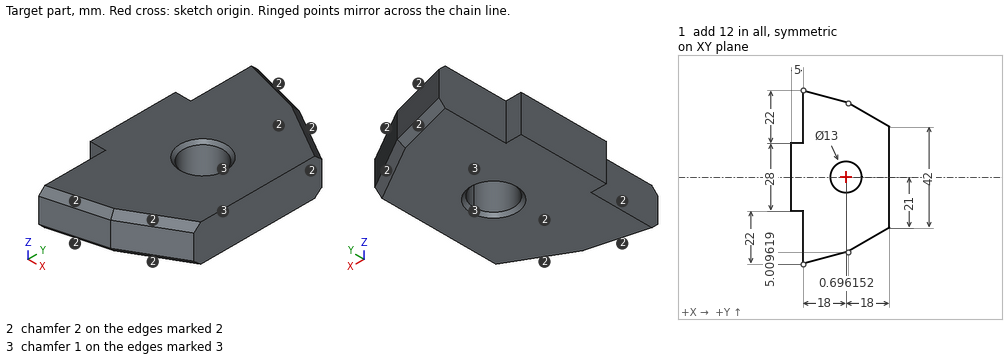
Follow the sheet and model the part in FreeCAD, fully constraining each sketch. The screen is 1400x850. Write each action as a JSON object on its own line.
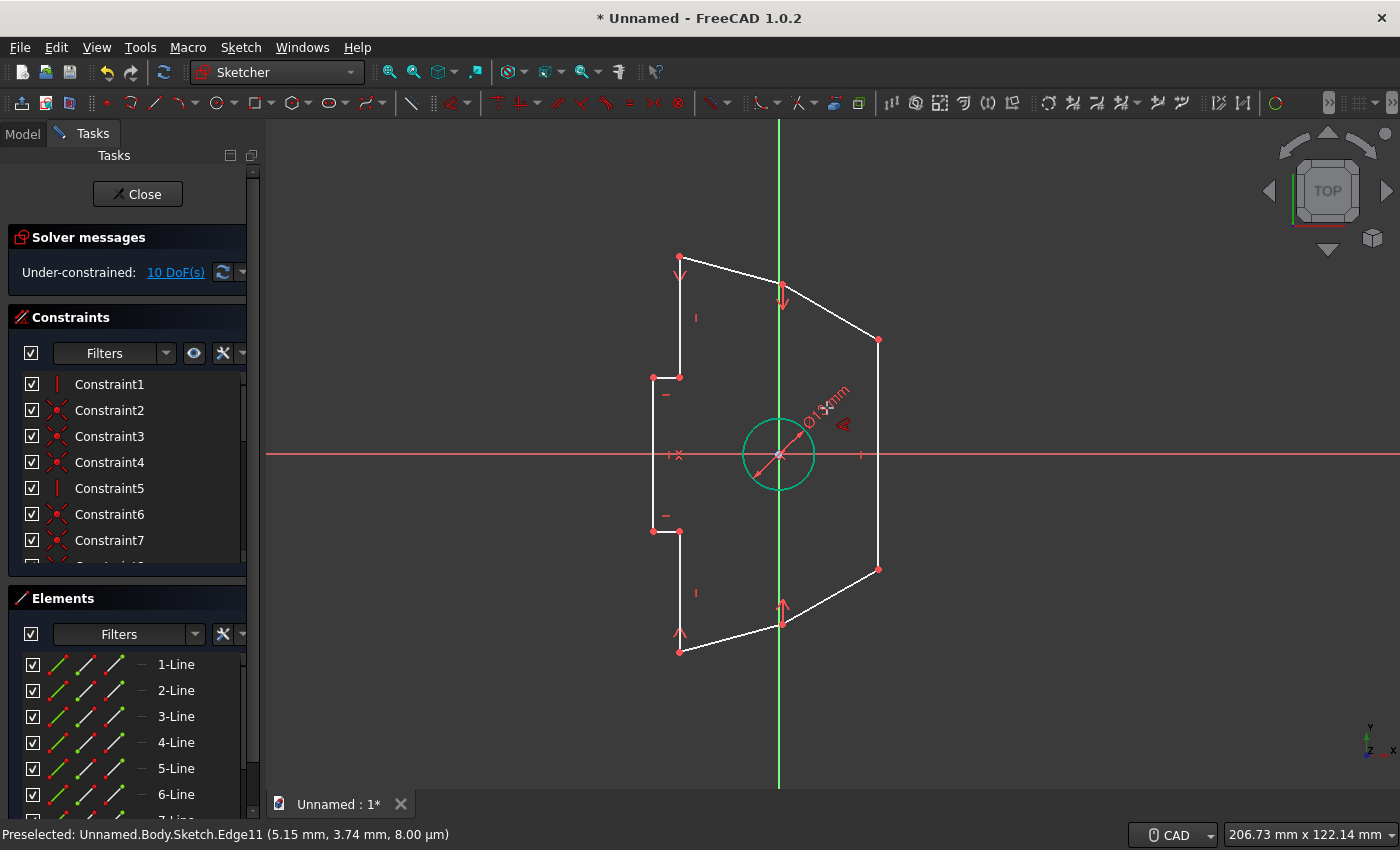
{"action": "scroll", "coordinate": [669, 378], "scroll_direction": "up", "scroll_amount": 2}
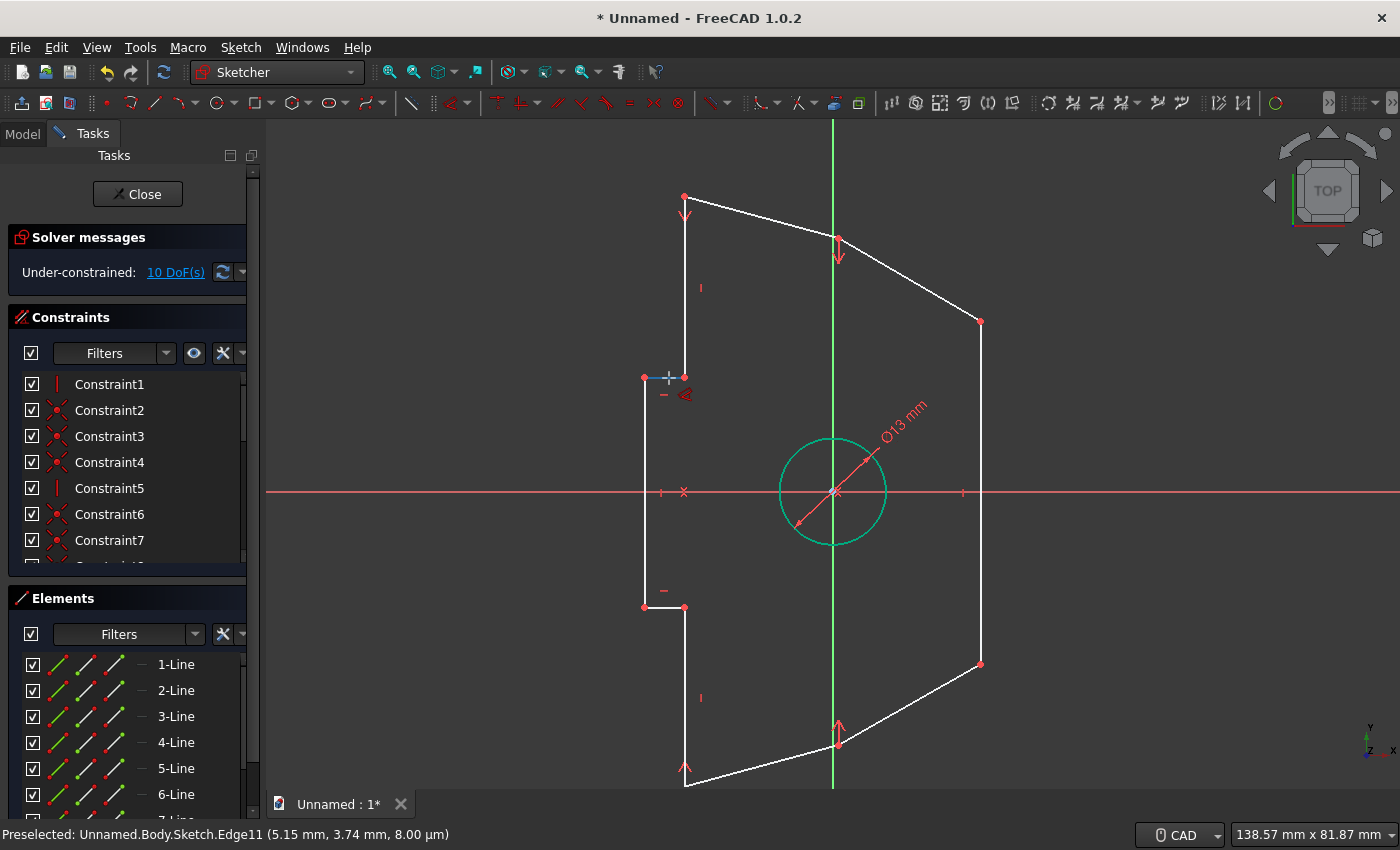
{"action": "left_click", "coordinate": [669, 378]}
{"action": "left_click", "coordinate": [665, 344]}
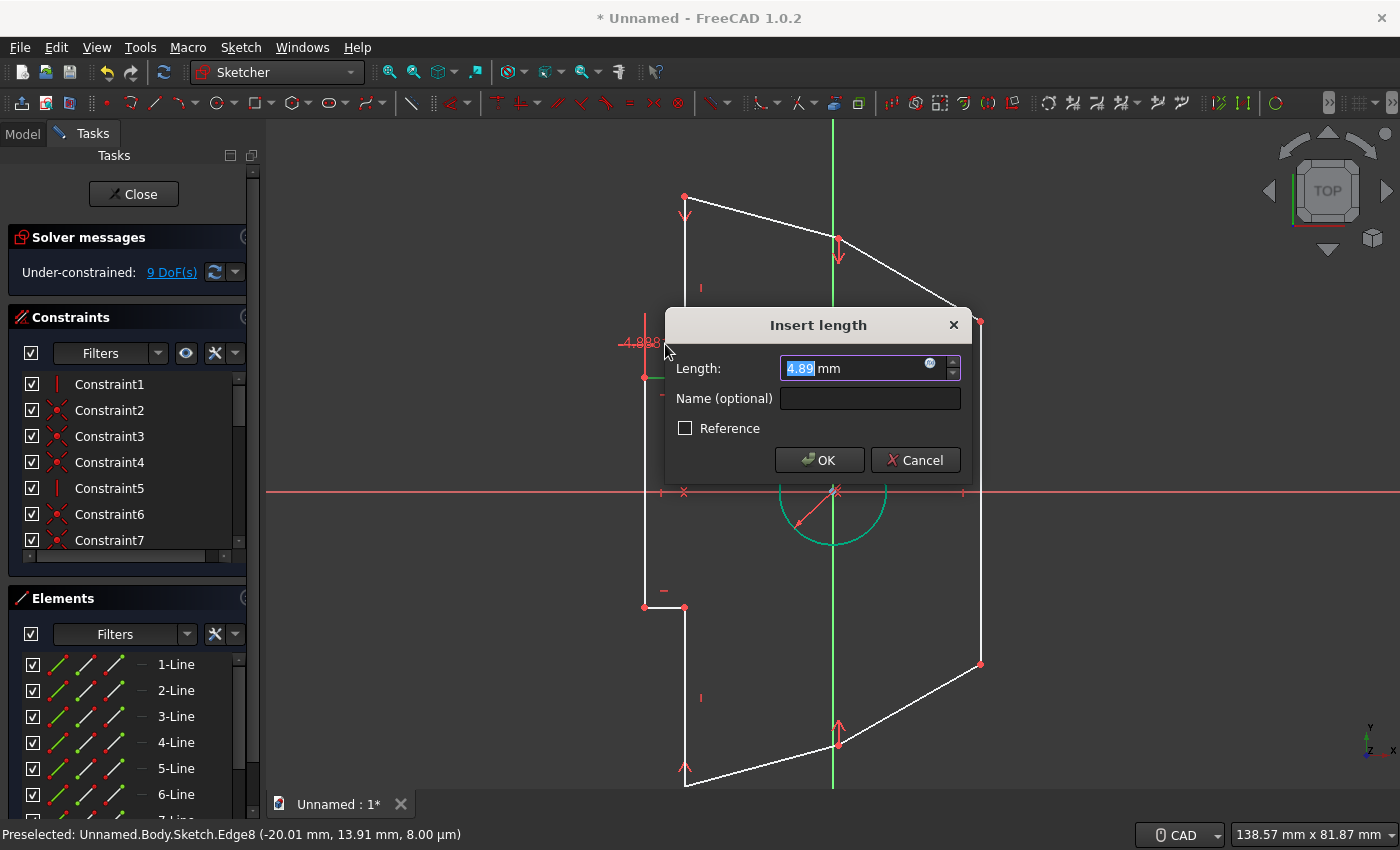
{"action": "type", "text": "5"}
{"action": "key", "text": "Return"}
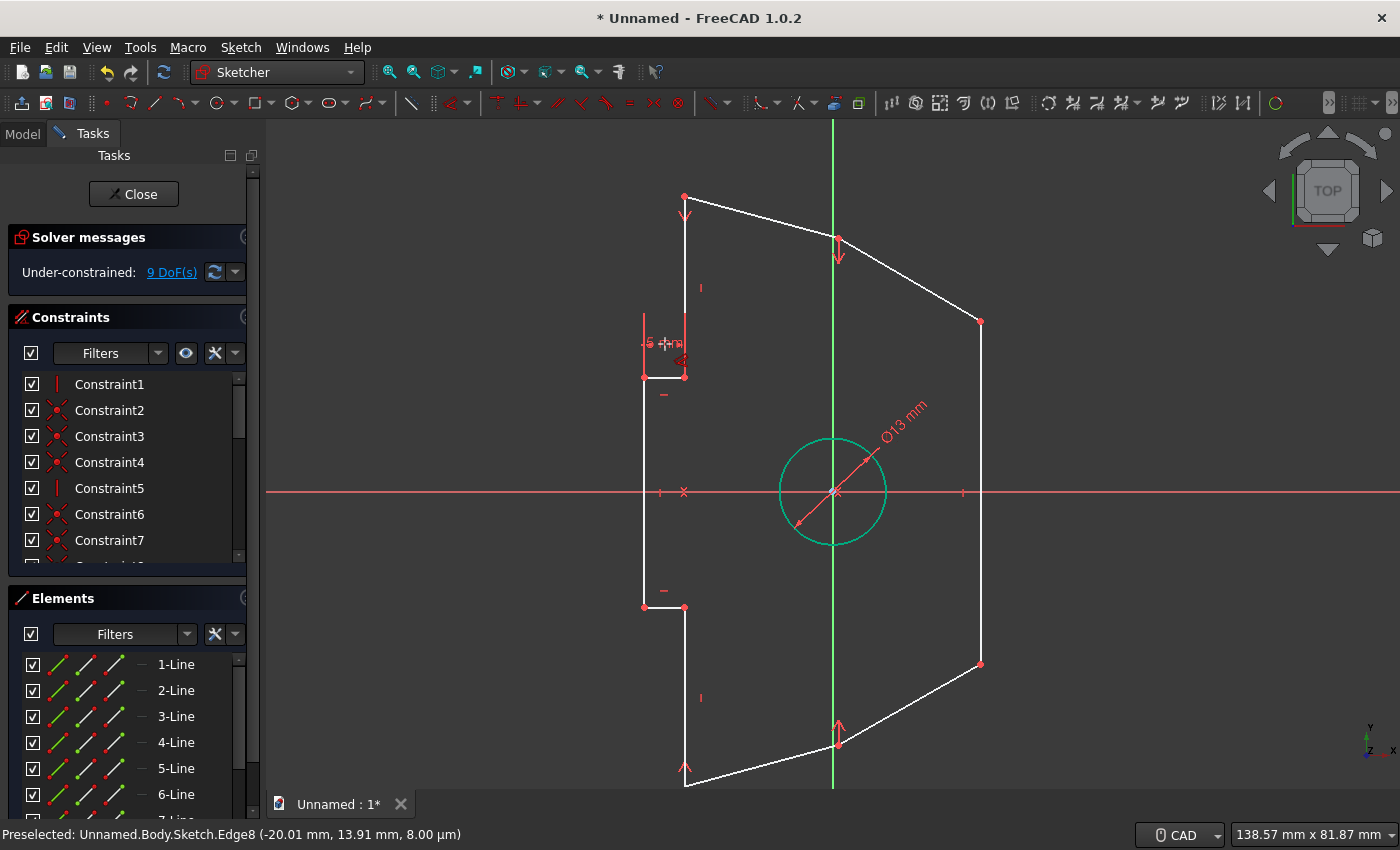
{"action": "left_click", "coordinate": [685, 661]}
{"action": "left_click", "coordinate": [651, 684]}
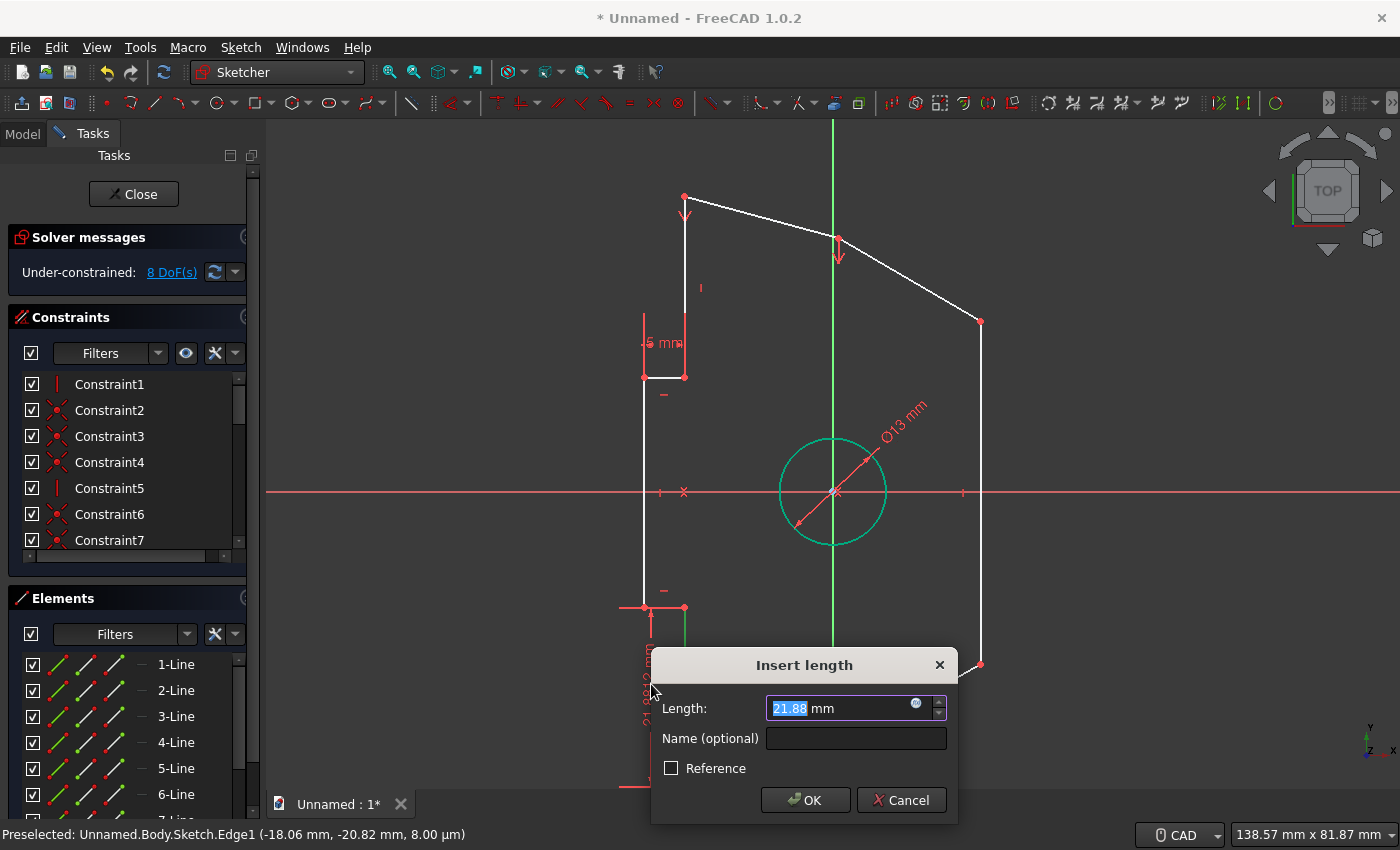
{"action": "type", "text": "22"}
{"action": "key", "text": "Return"}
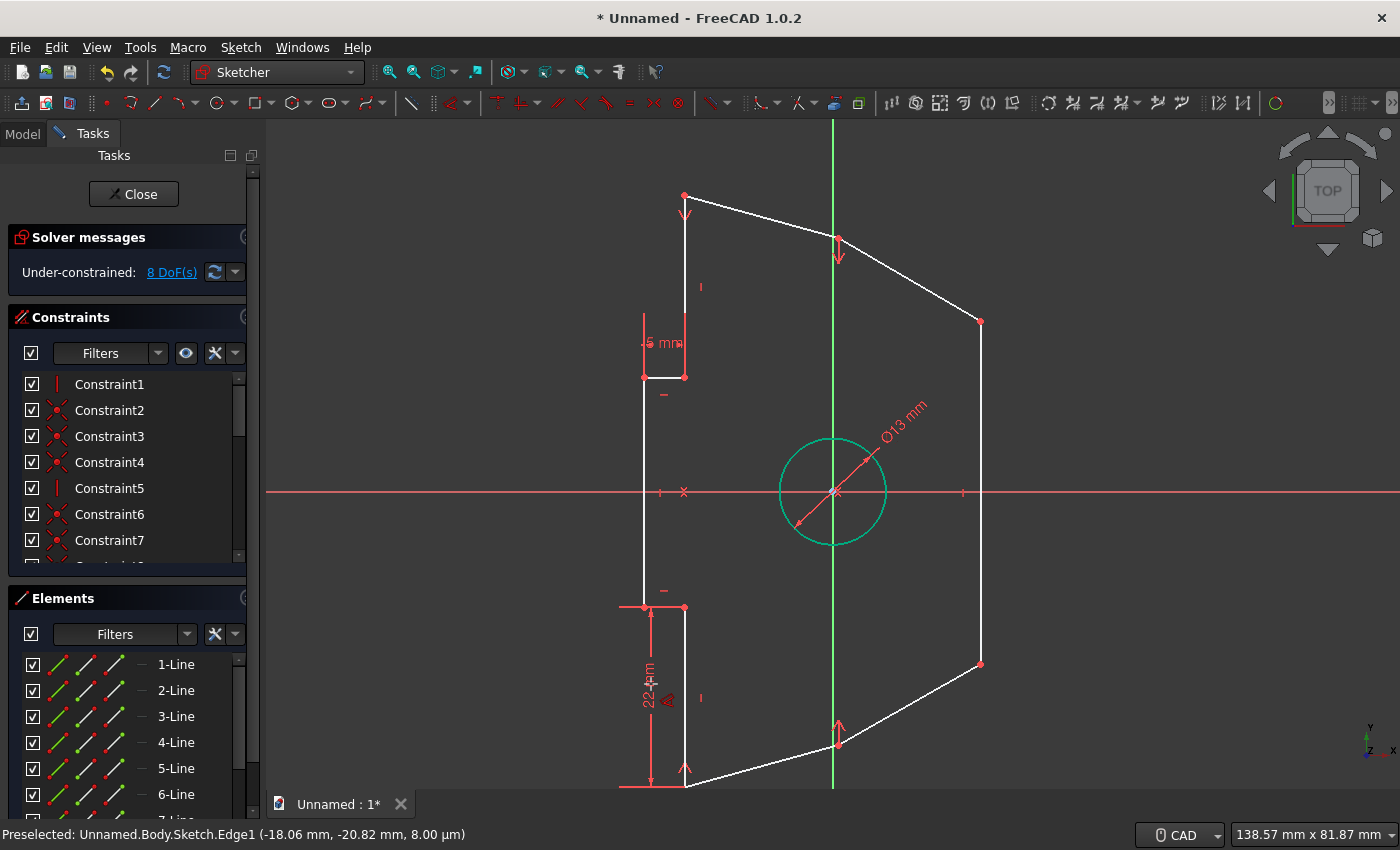
{"action": "left_click", "coordinate": [981, 561]}
{"action": "left_click", "coordinate": [1015, 414]}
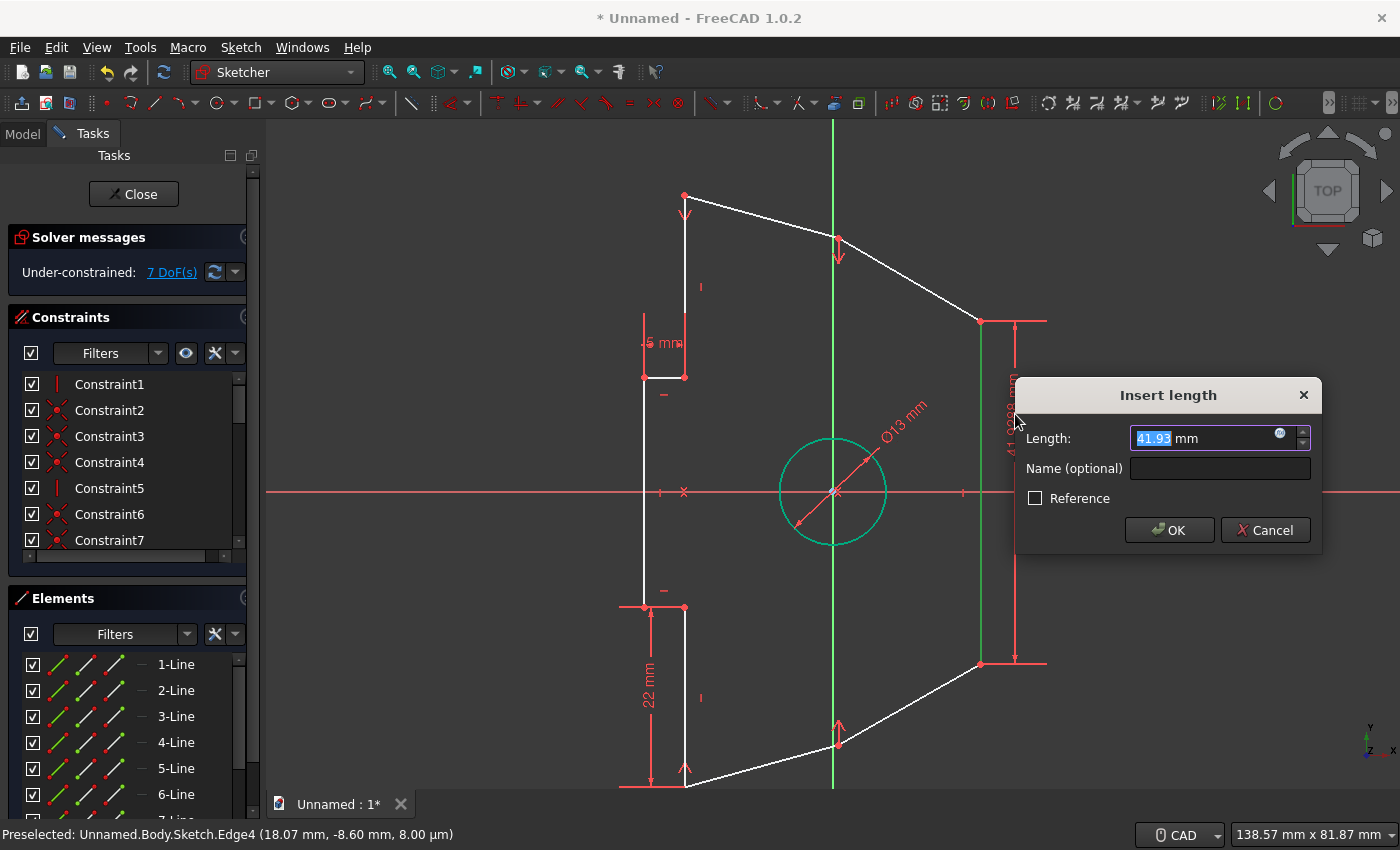
{"action": "type", "text": "42"}
{"action": "key", "text": "Return"}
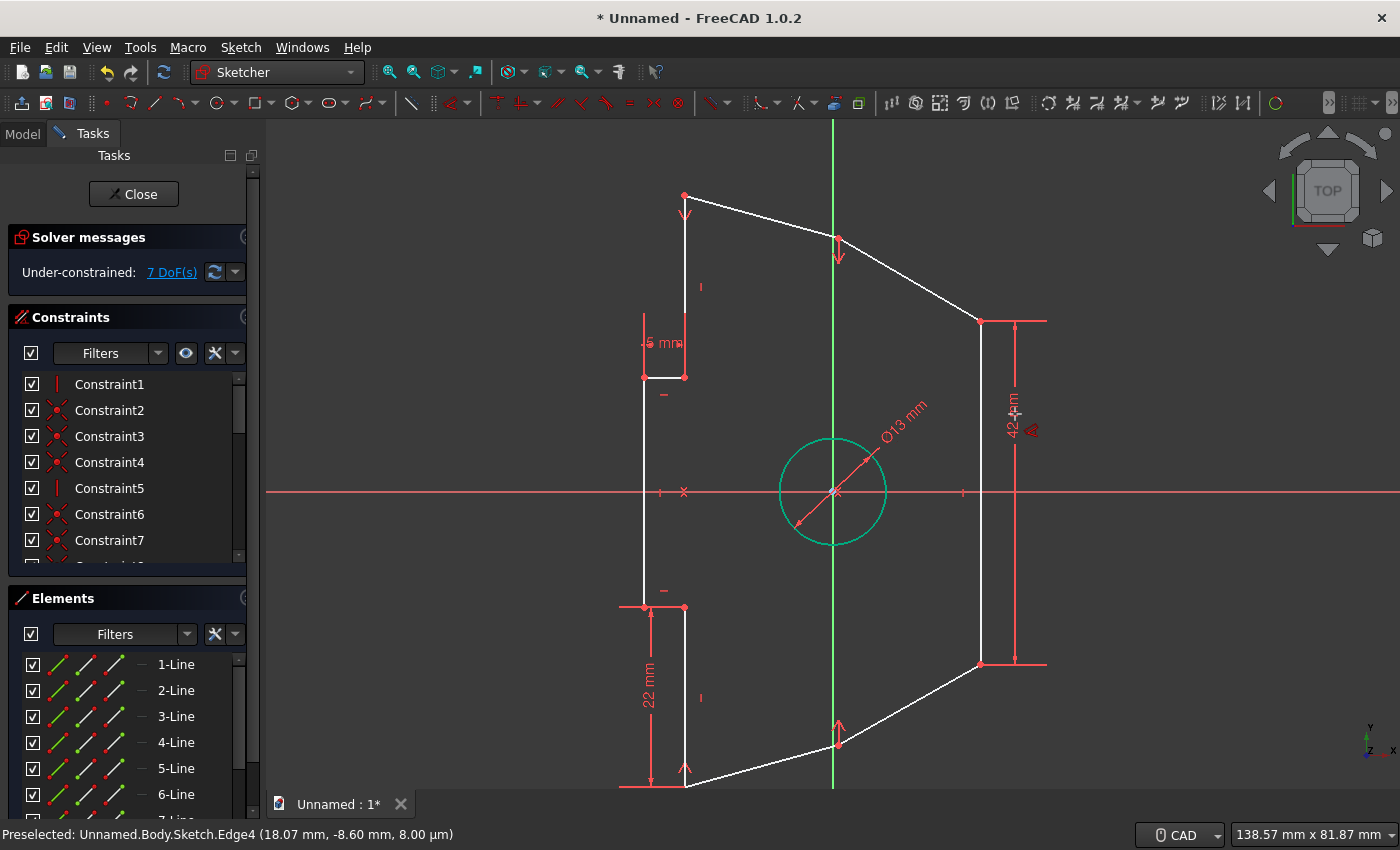
{"action": "left_click", "coordinate": [685, 250]}
{"action": "left_click", "coordinate": [651, 287]}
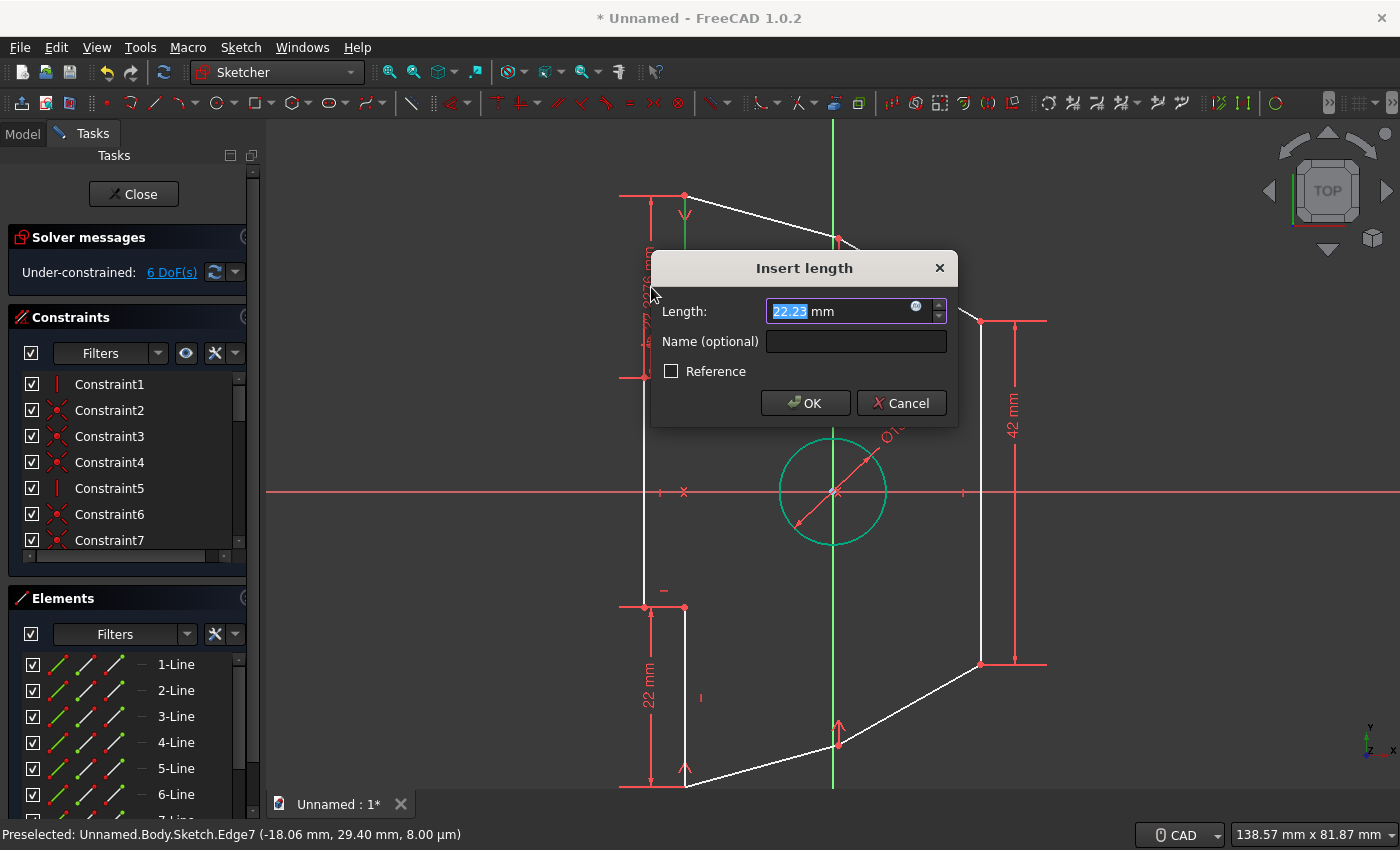
{"action": "type", "text": "22"}
{"action": "key", "text": "Return"}